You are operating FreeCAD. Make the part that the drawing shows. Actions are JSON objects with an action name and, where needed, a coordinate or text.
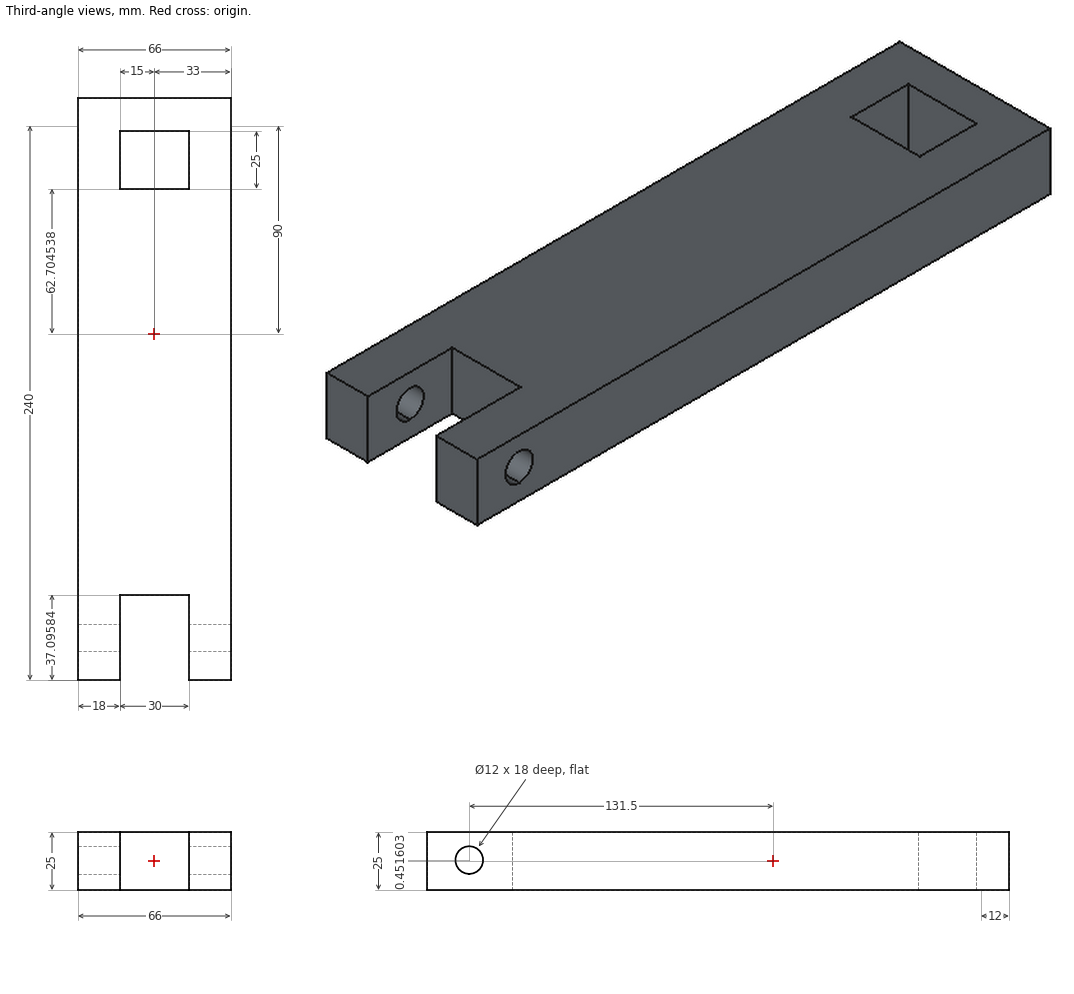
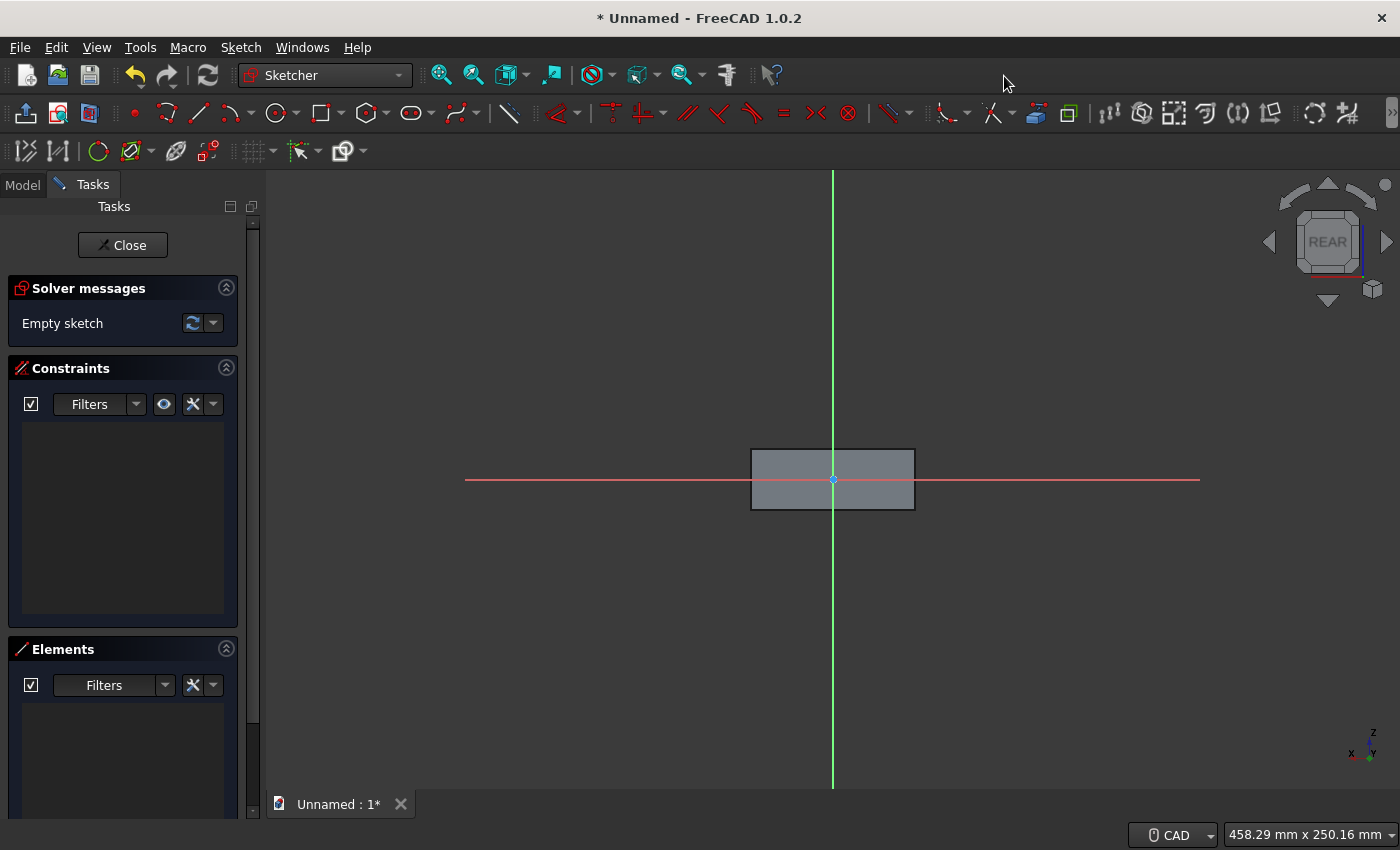
{"action": "scroll", "coordinate": [855, 480], "scroll_direction": "up", "scroll_amount": 7}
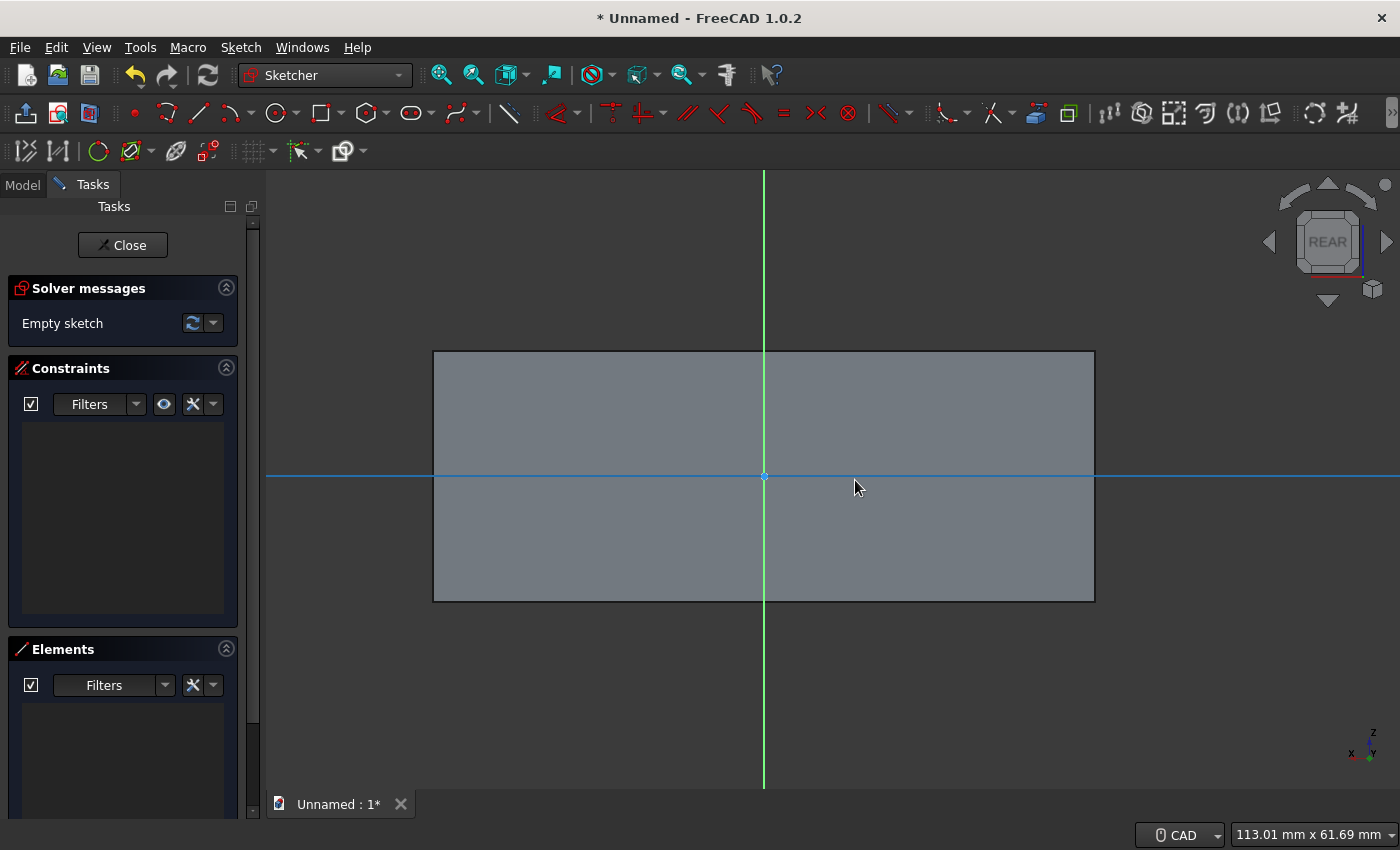
{"action": "key", "text": "g v"}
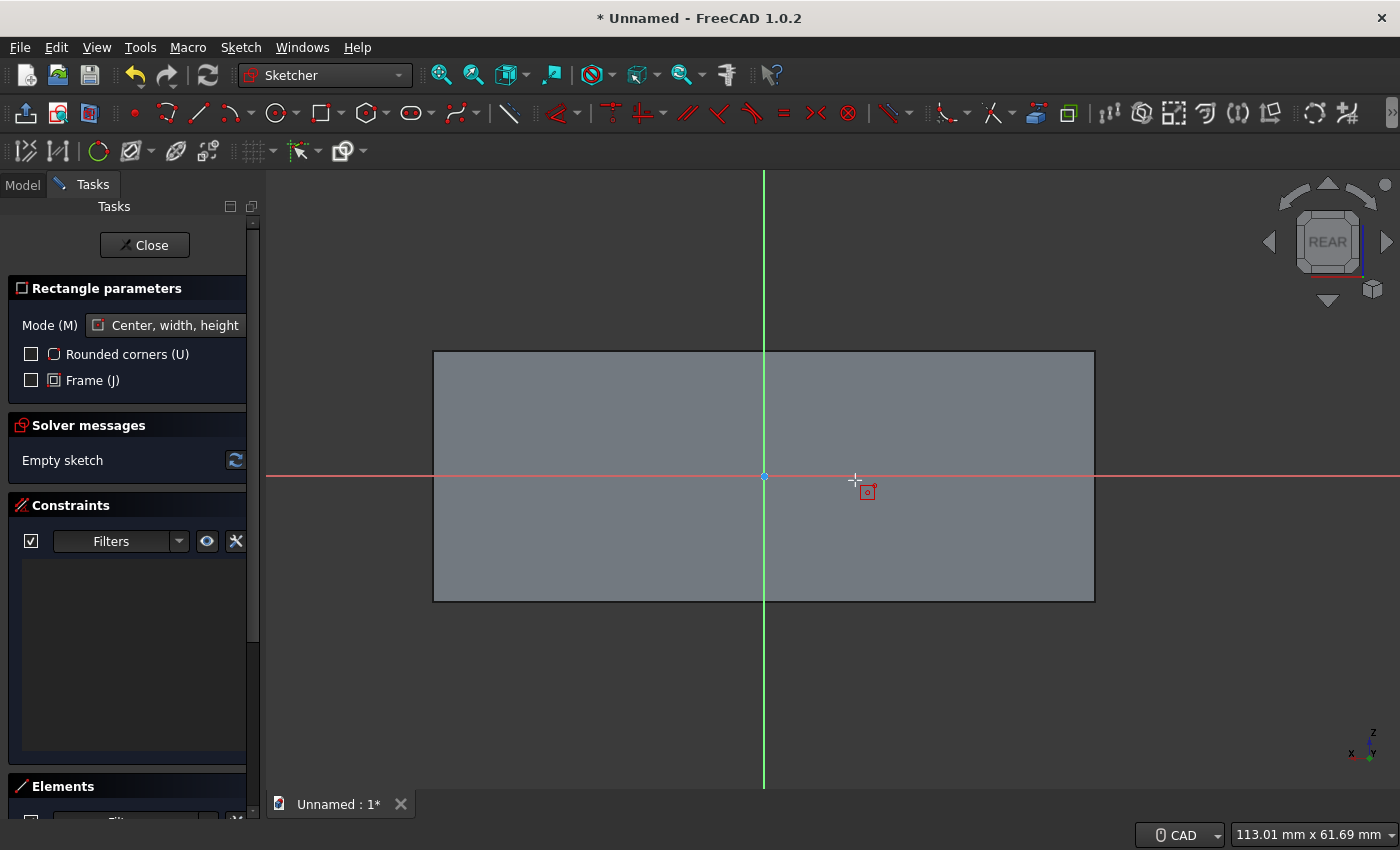
{"action": "left_click", "coordinate": [764, 476]}
{"action": "mouse_move", "coordinate": [1095, 351]}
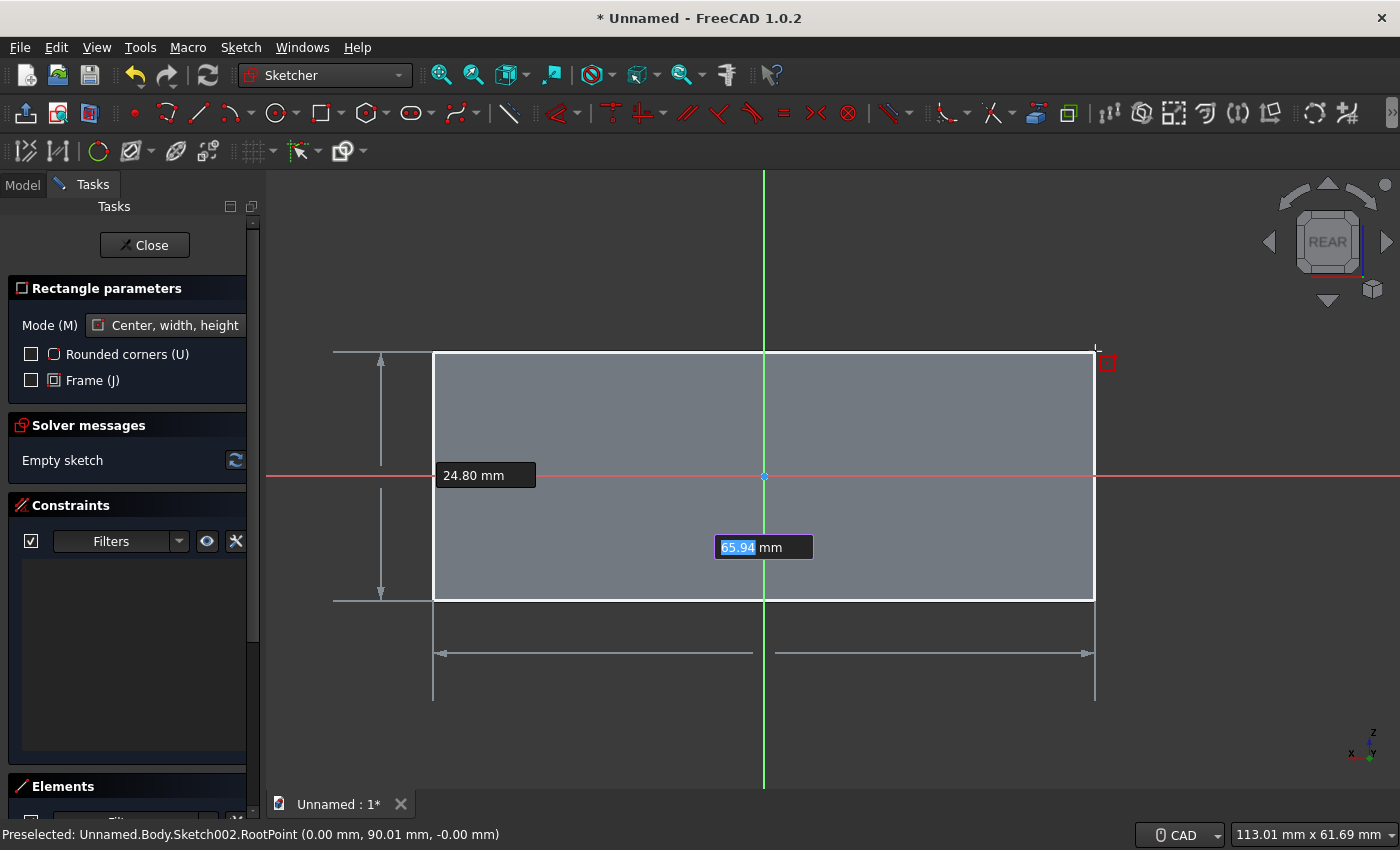
{"action": "type", "text": "66"}
{"action": "key", "text": "Tab"}
{"action": "type", "text": "25"}
{"action": "key", "text": "Return"}
{"action": "key", "text": "Escape"}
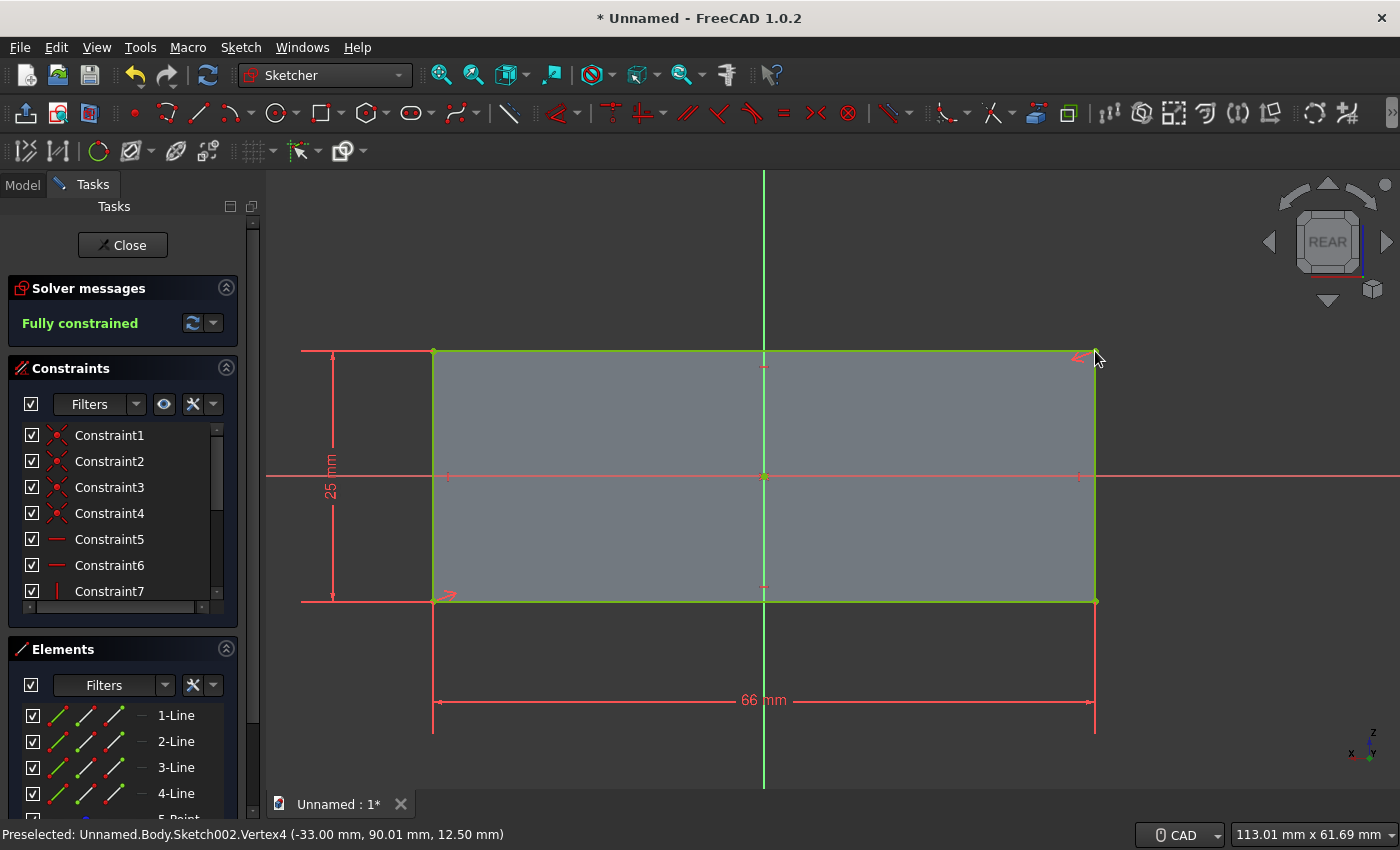
{"action": "left_click", "coordinate": [123, 245]}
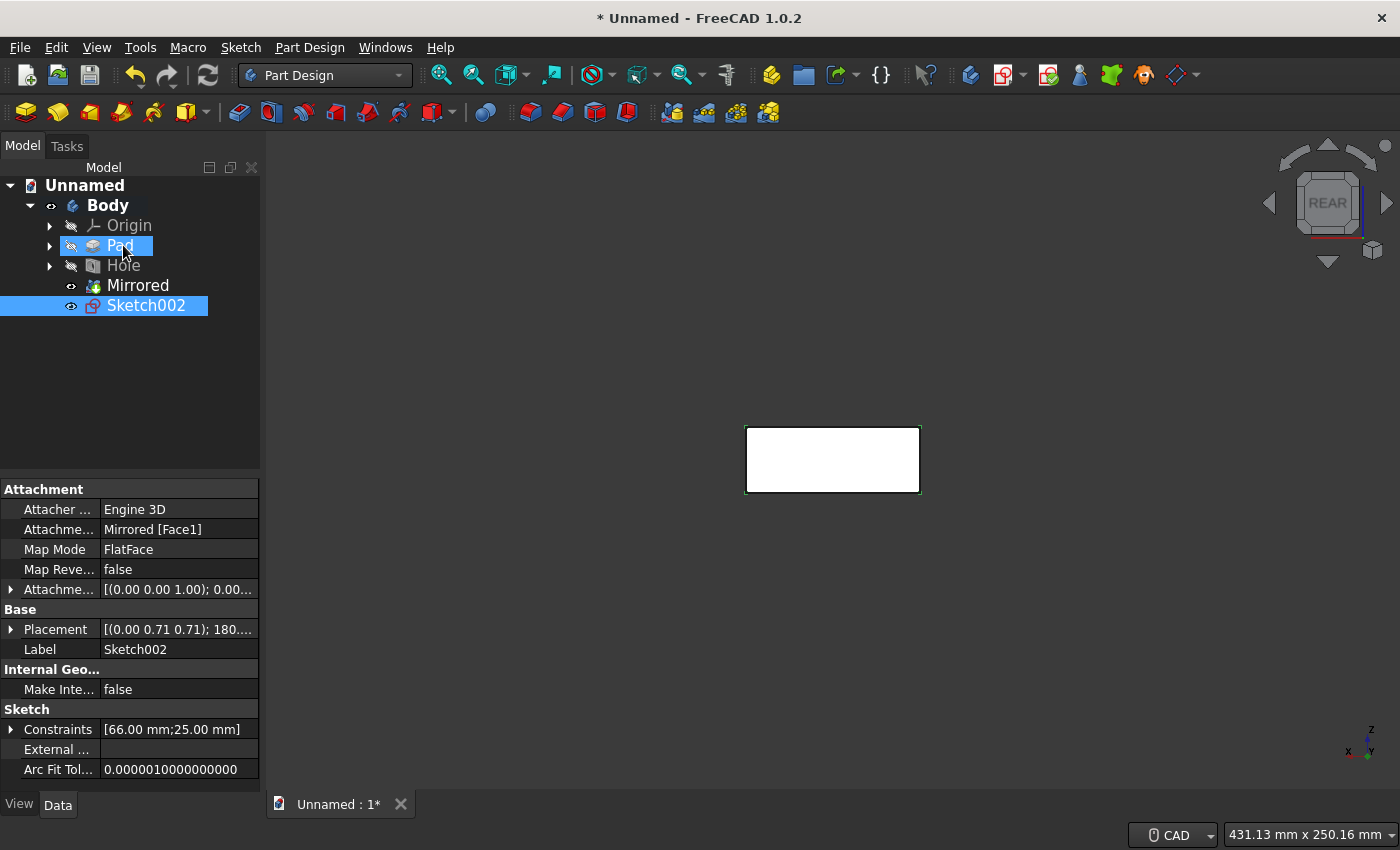
{"action": "left_click", "coordinate": [26, 112]}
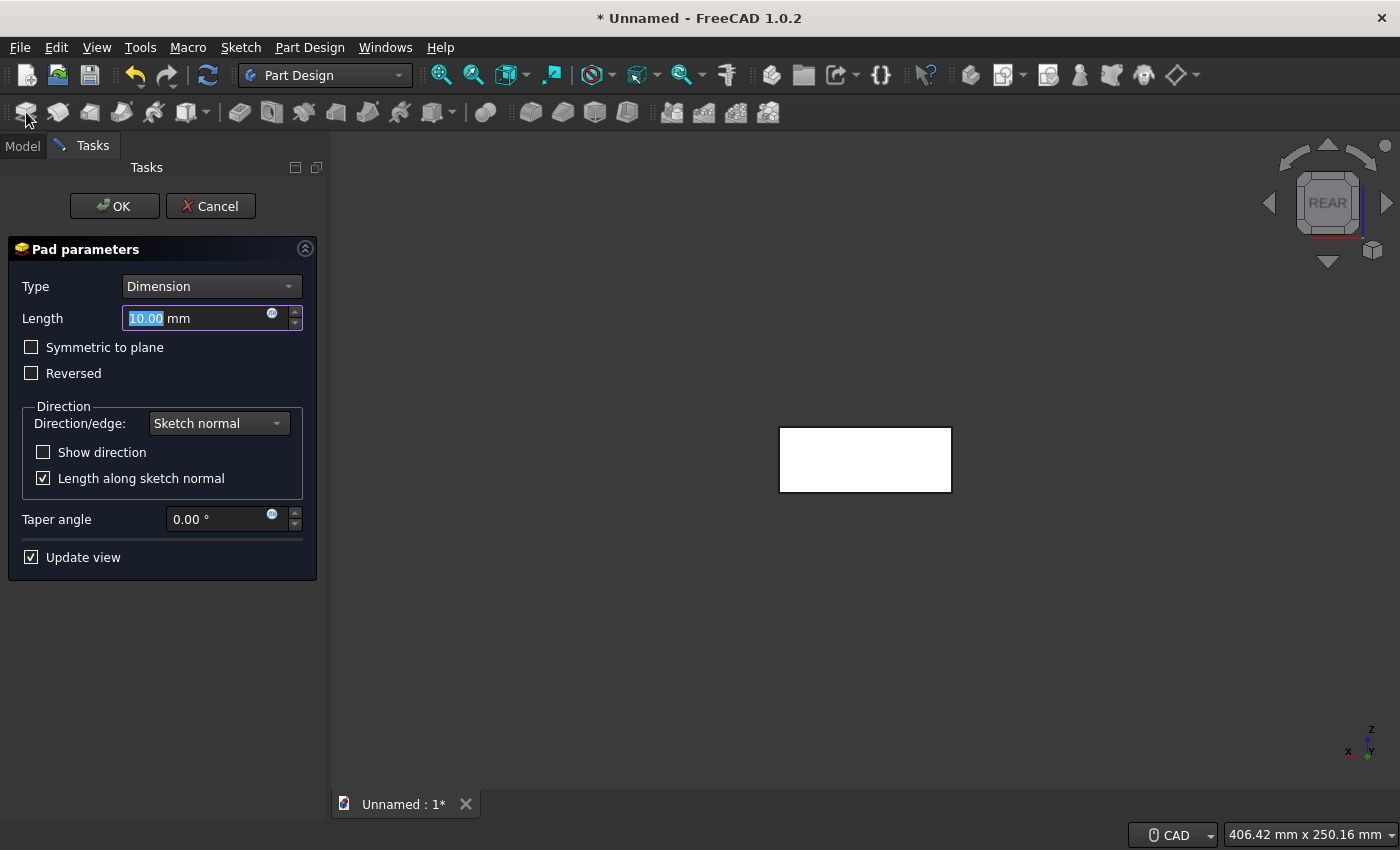
{"action": "type", "text": "12"}
{"action": "key", "text": "Tab"}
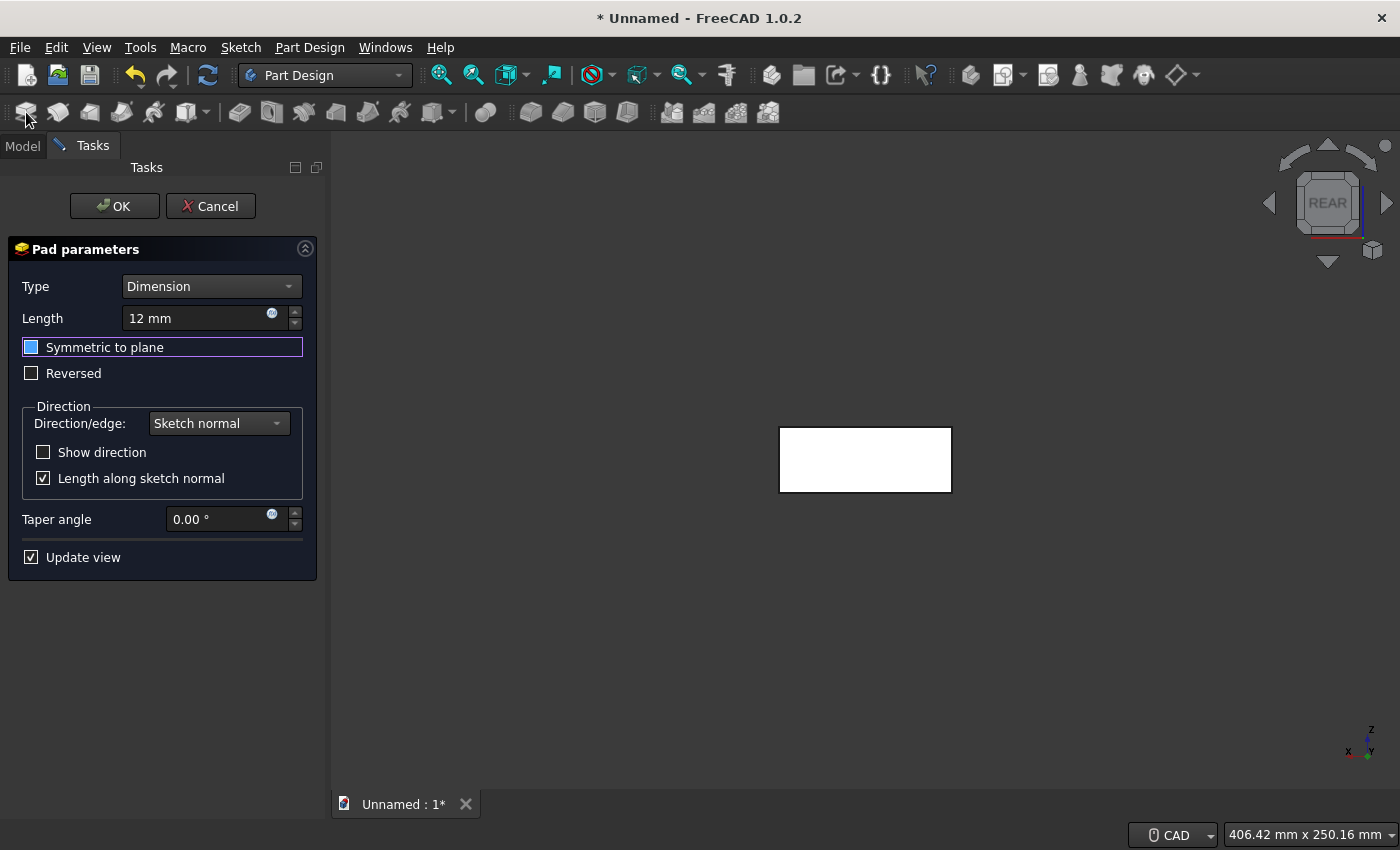
{"action": "left_click", "coordinate": [115, 206]}